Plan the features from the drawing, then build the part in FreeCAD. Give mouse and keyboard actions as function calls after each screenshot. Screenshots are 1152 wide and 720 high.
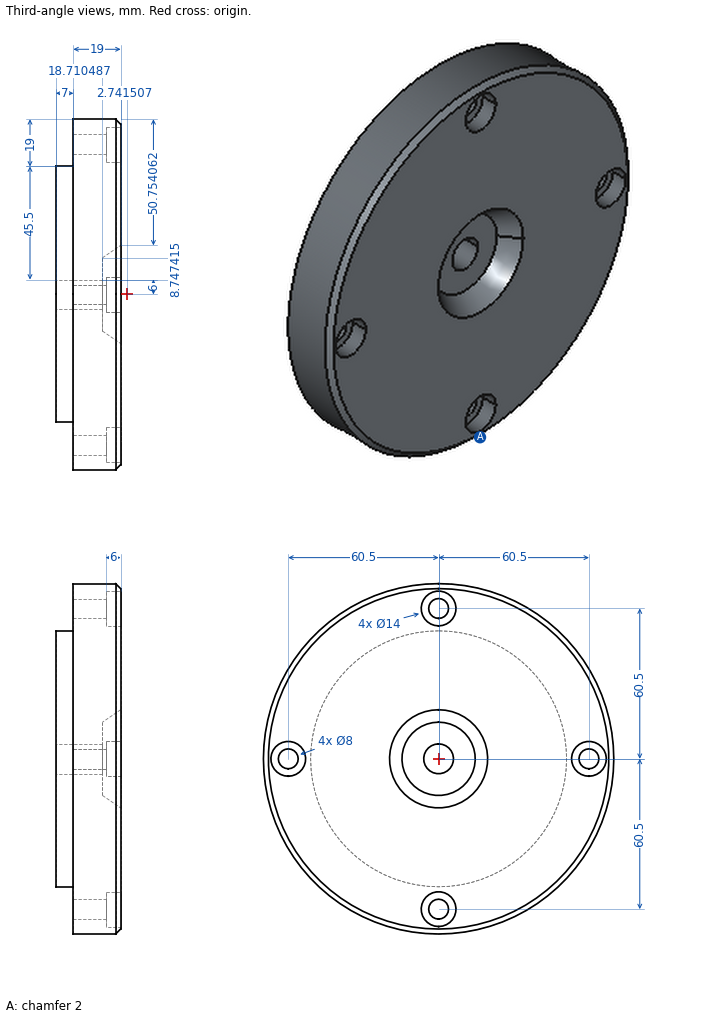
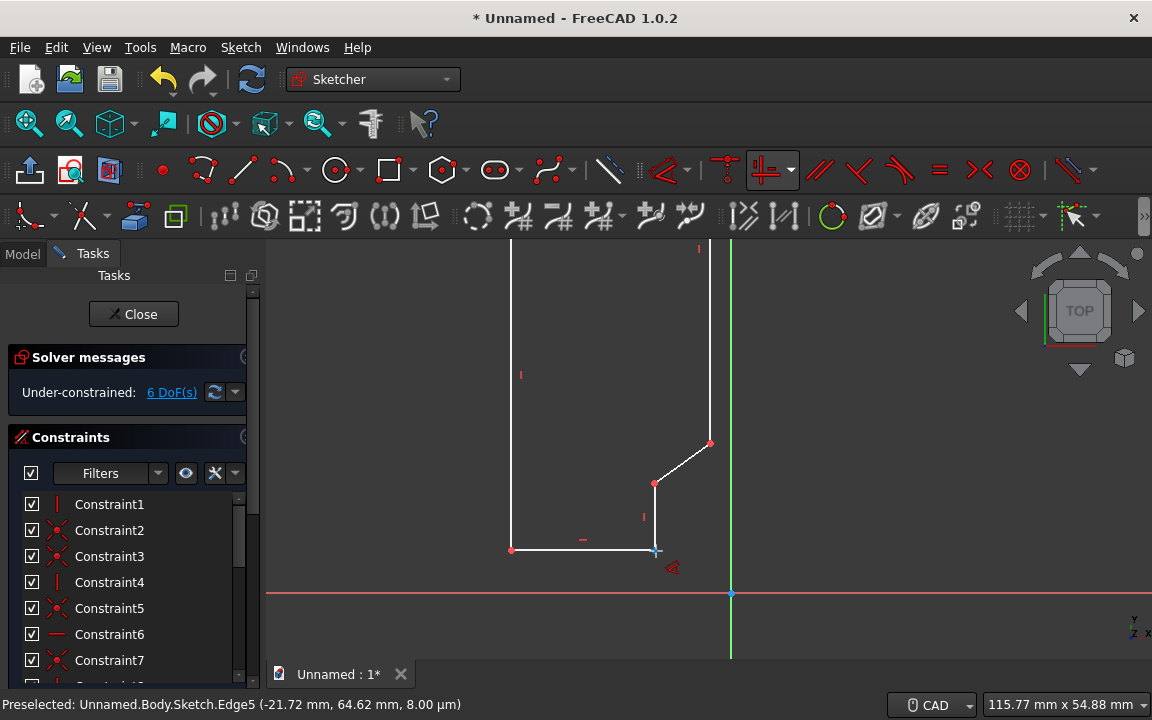
click(655, 550)
click(765, 572)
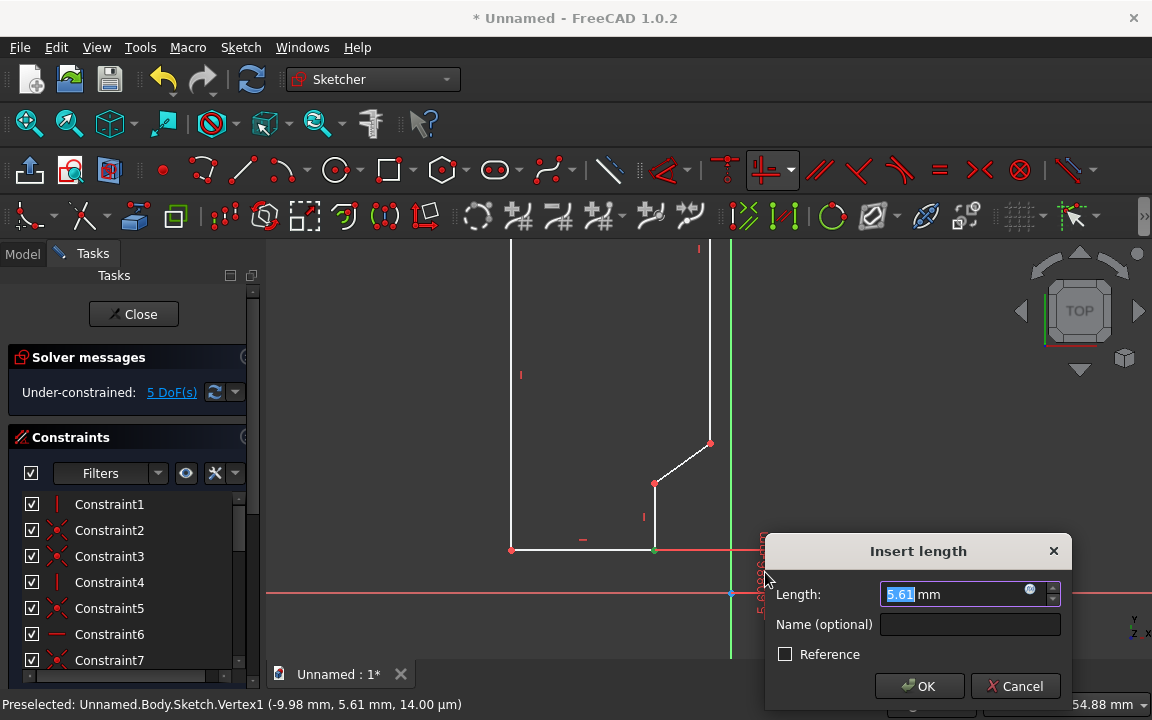
text(6)
key(Return)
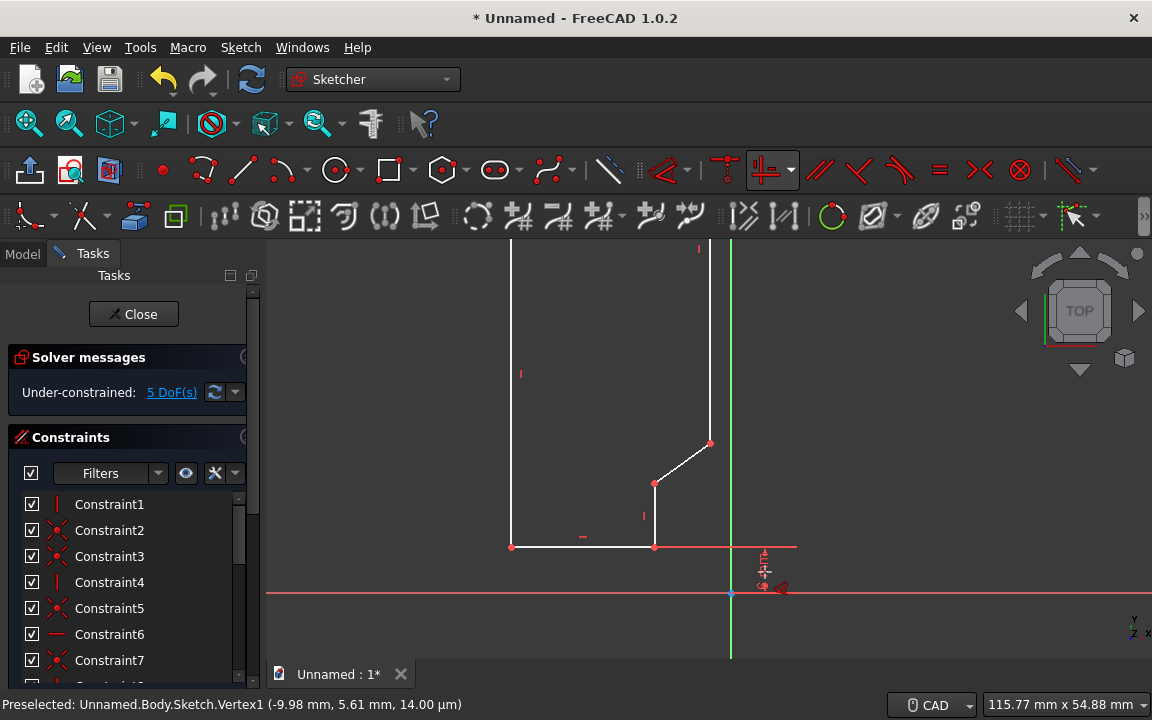
click(511, 304)
click(477, 407)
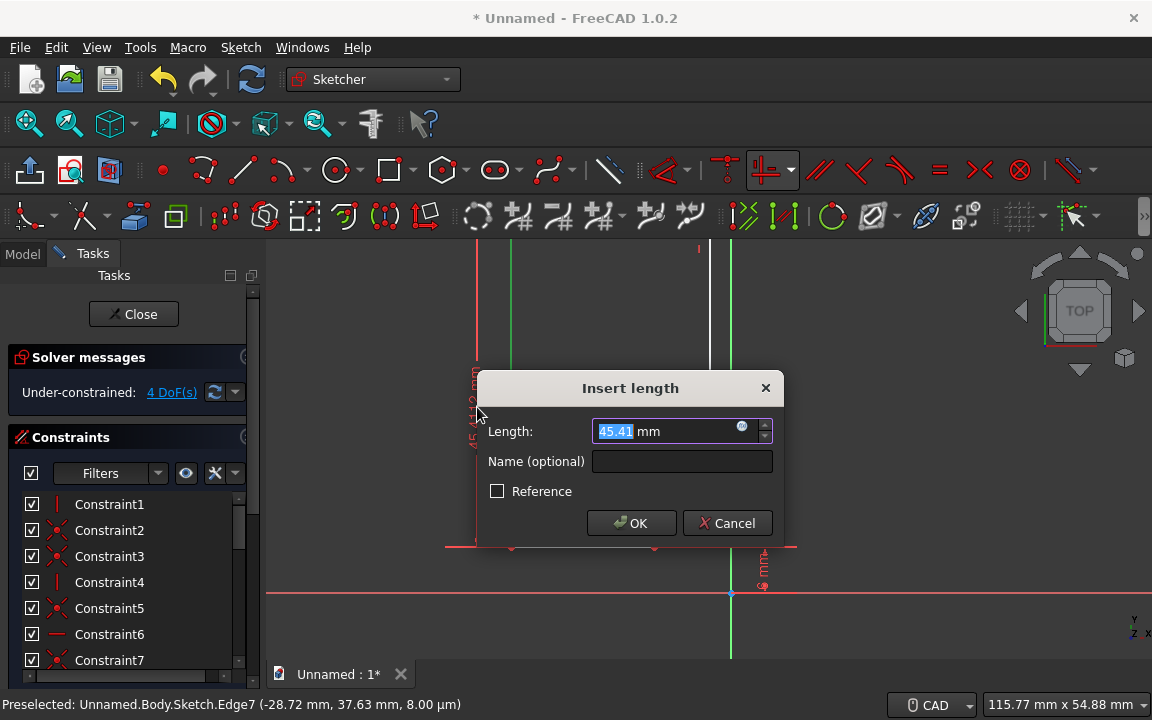
text(45.5)
key(Return)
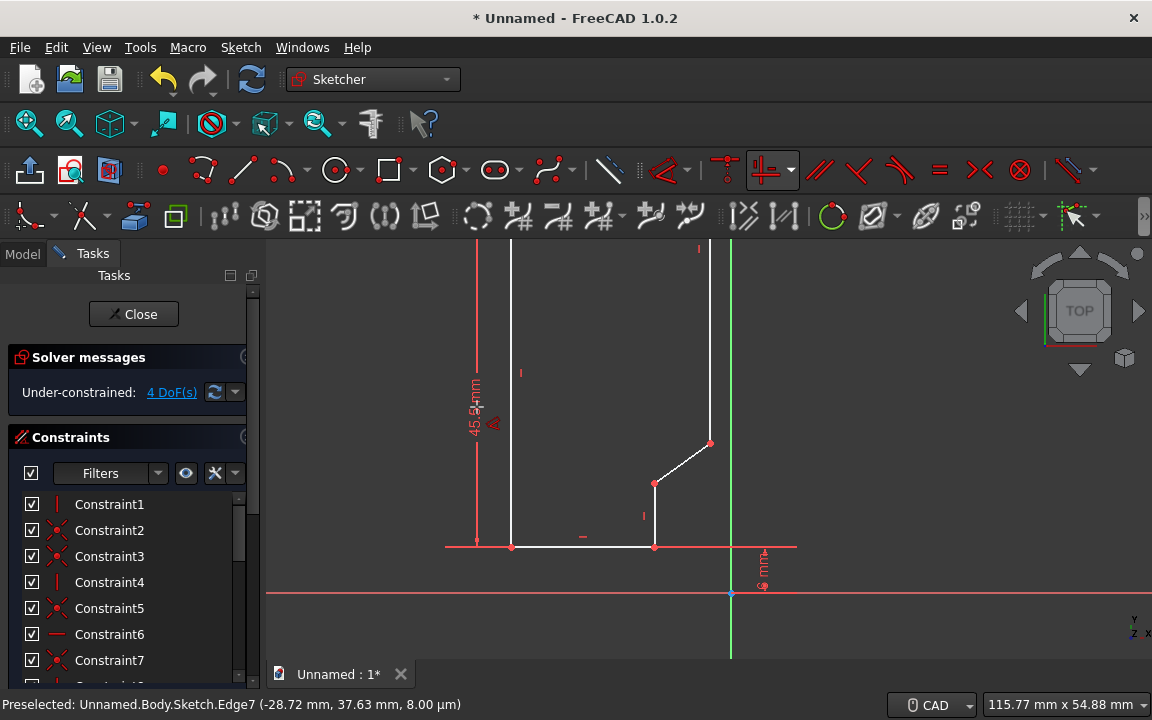
click(655, 528)
click(689, 515)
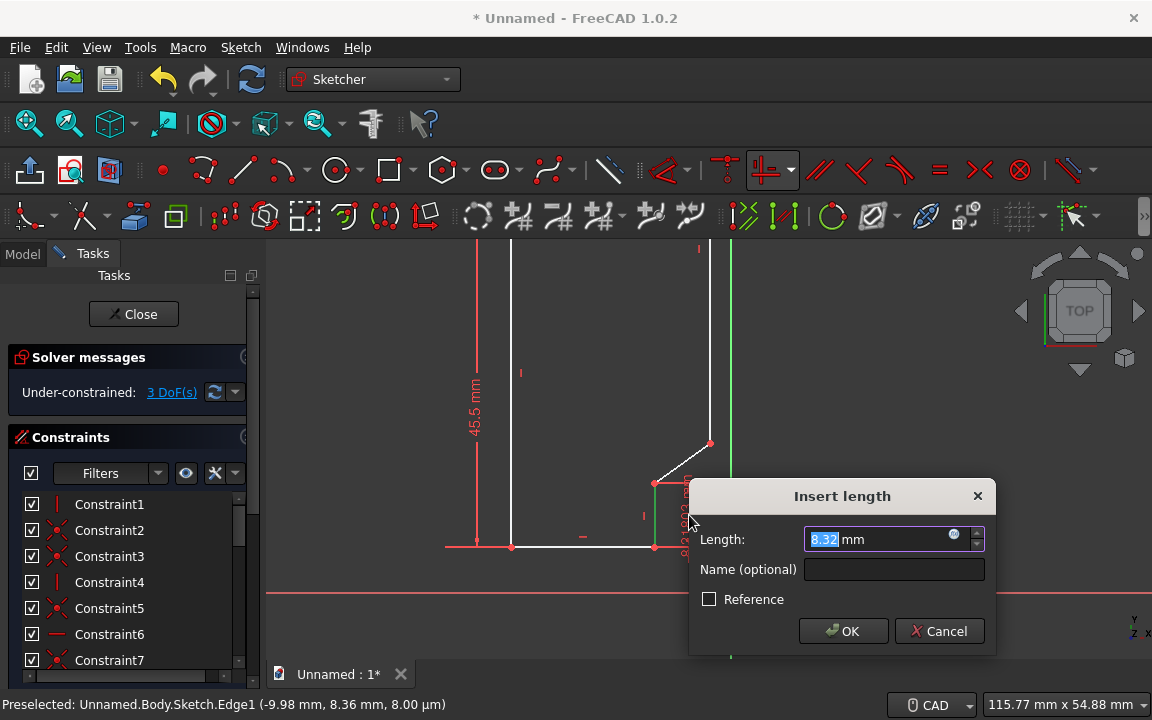
text(8.747415)
key(Return)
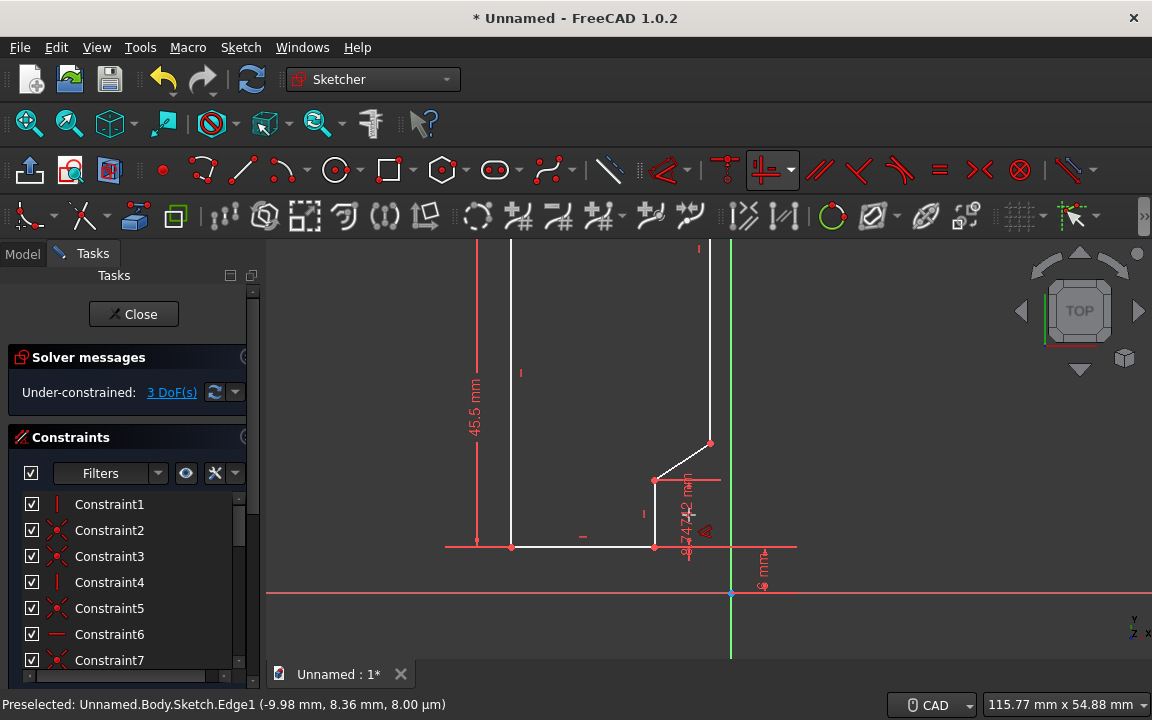
click(710, 326)
click(744, 355)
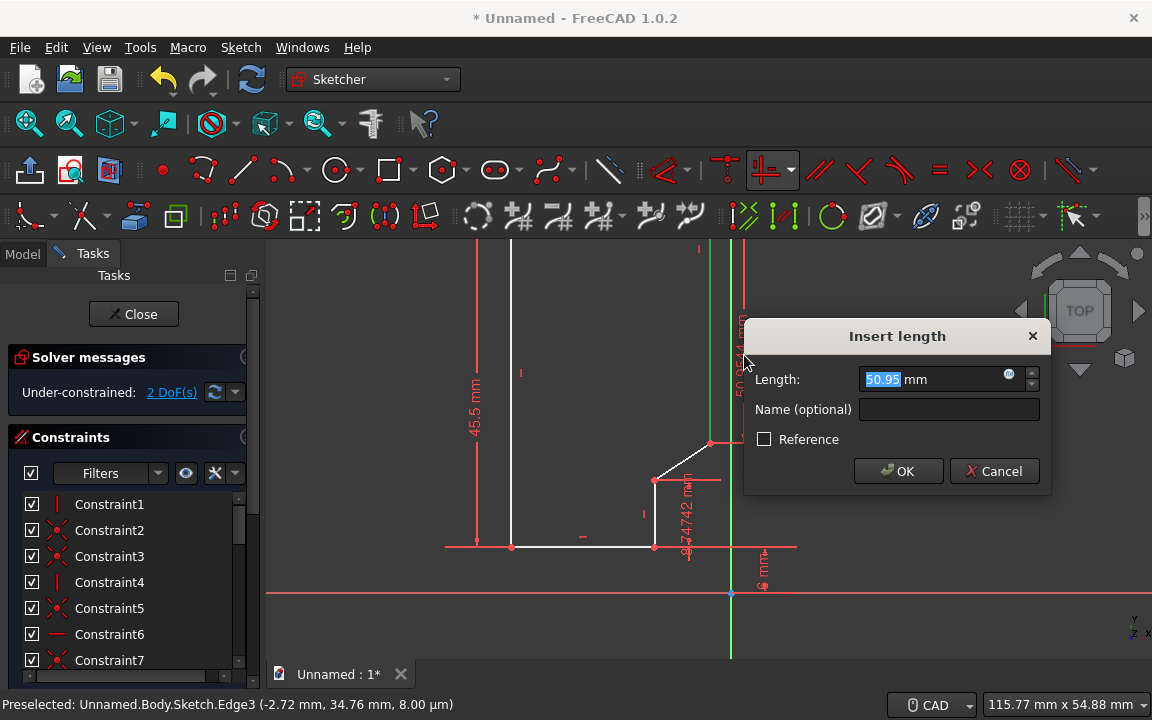
text(50.754062)
key(Return)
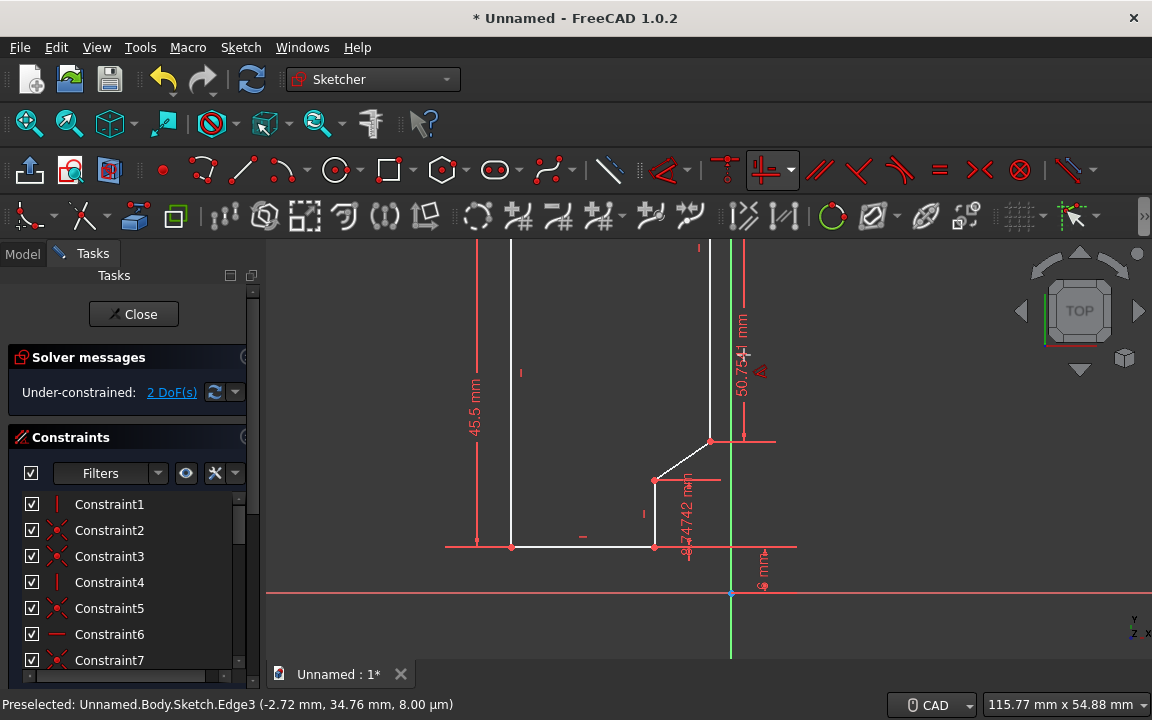
click(554, 547)
click(583, 513)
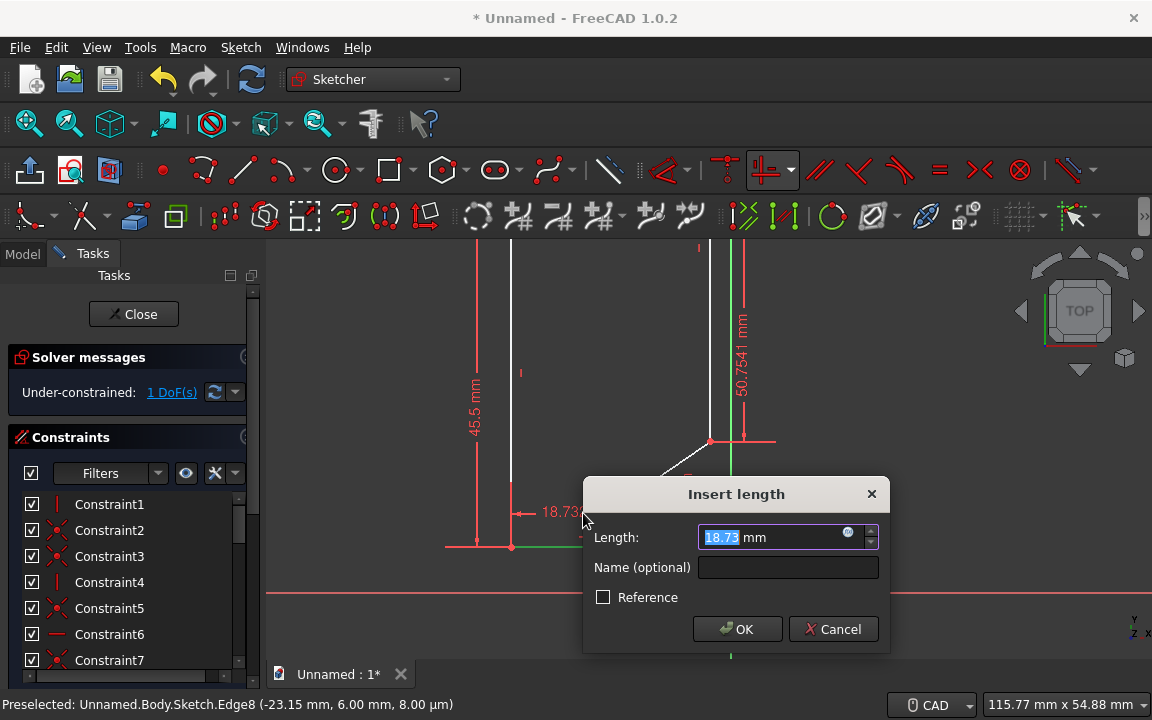
text(18.710487)
key(Return)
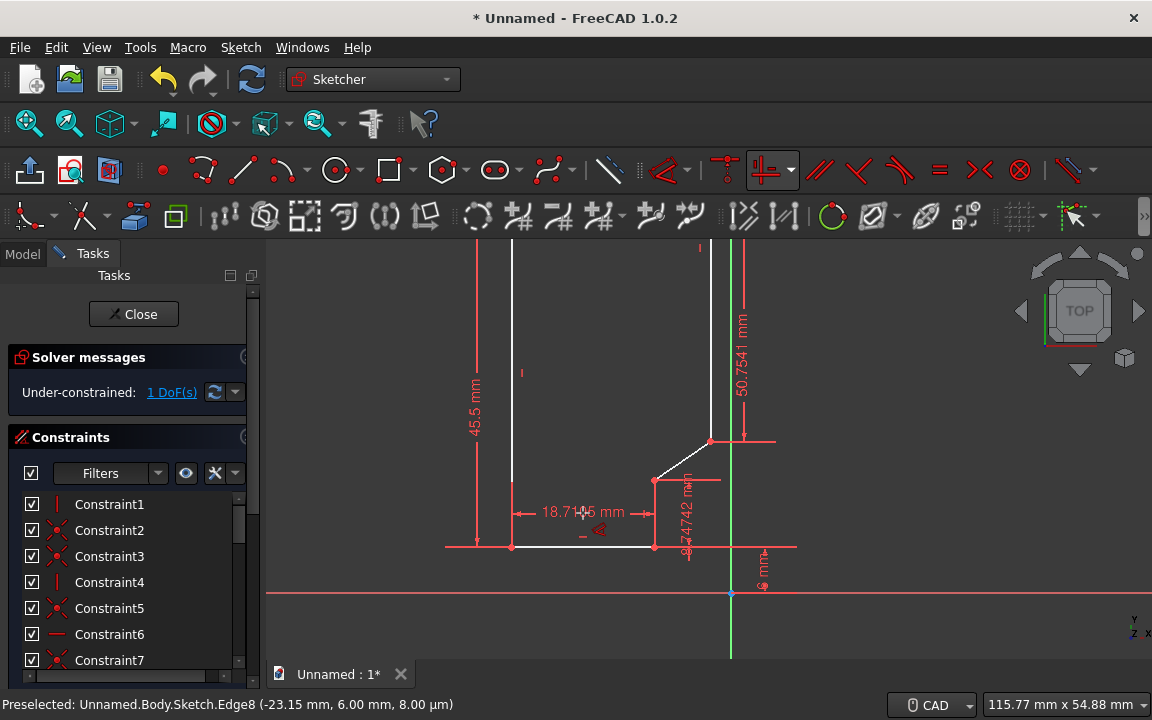
scroll(711, 442, up, 4)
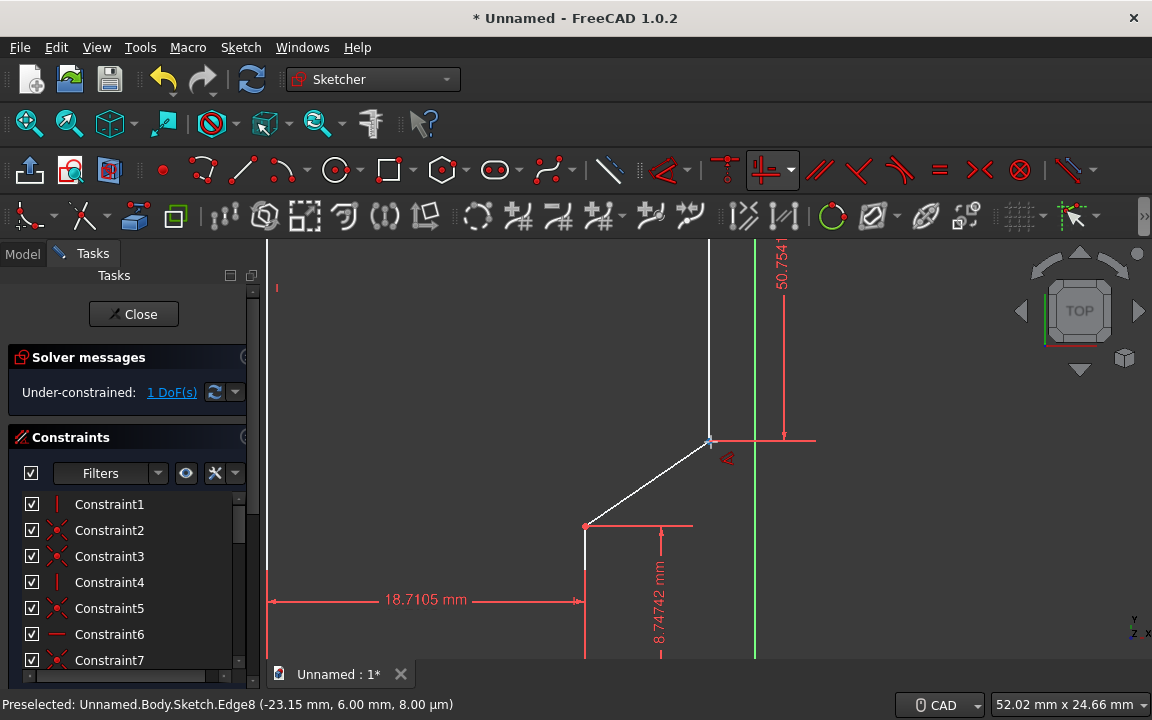
click(709, 441)
click(732, 407)